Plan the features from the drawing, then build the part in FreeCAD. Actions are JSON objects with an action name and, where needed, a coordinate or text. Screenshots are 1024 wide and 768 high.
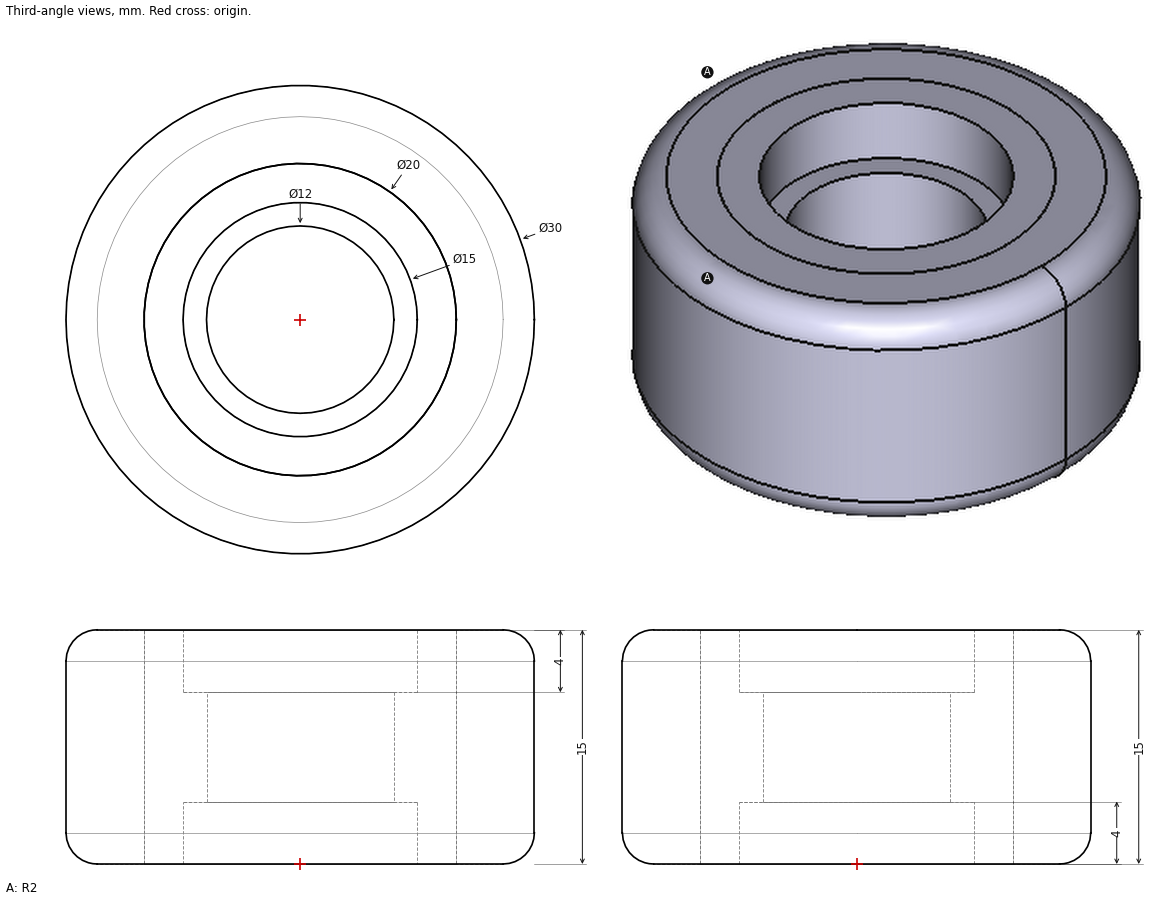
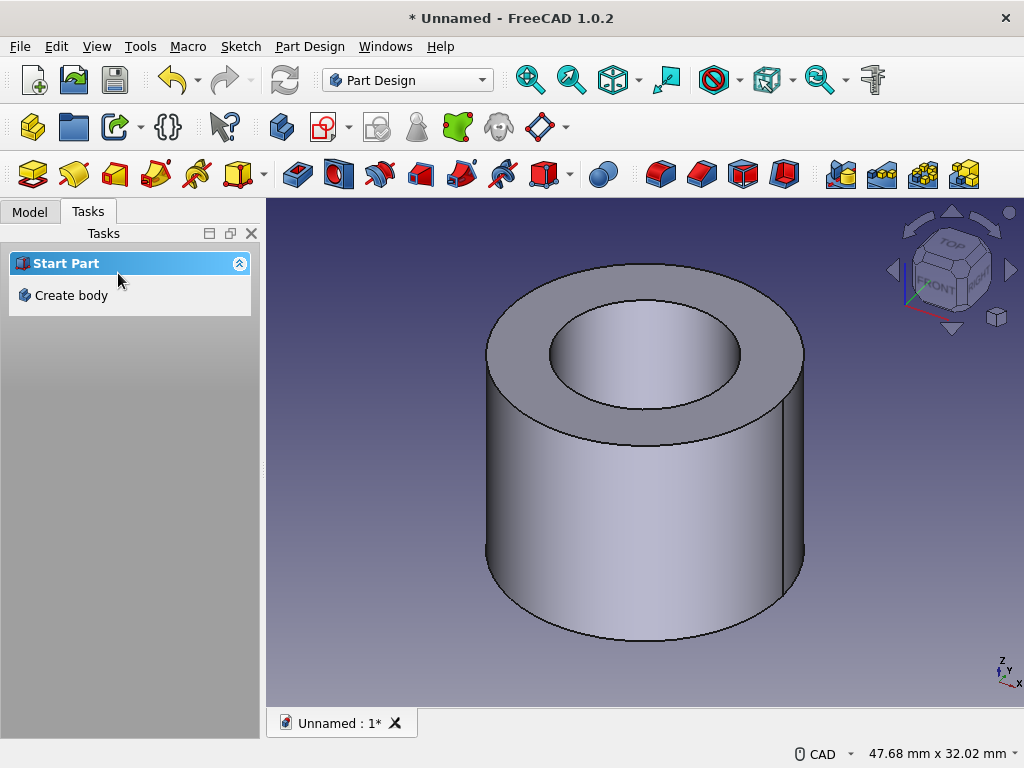
{"action": "left_click", "coordinate": [678, 425]}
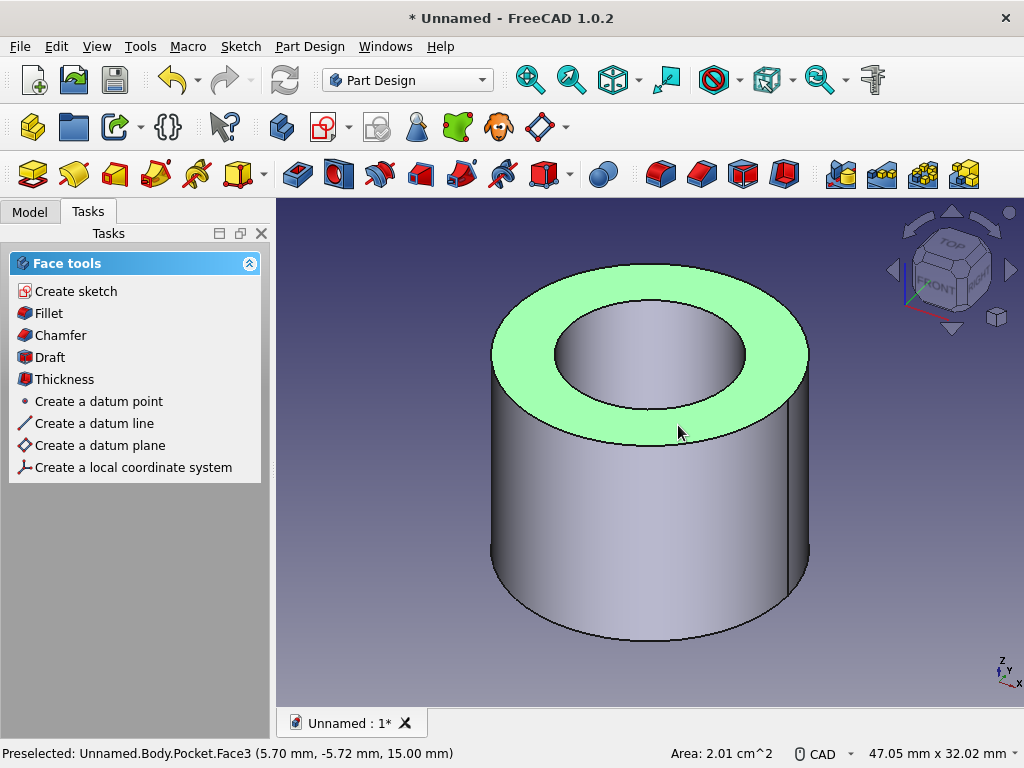
{"action": "left_click", "coordinate": [322, 128]}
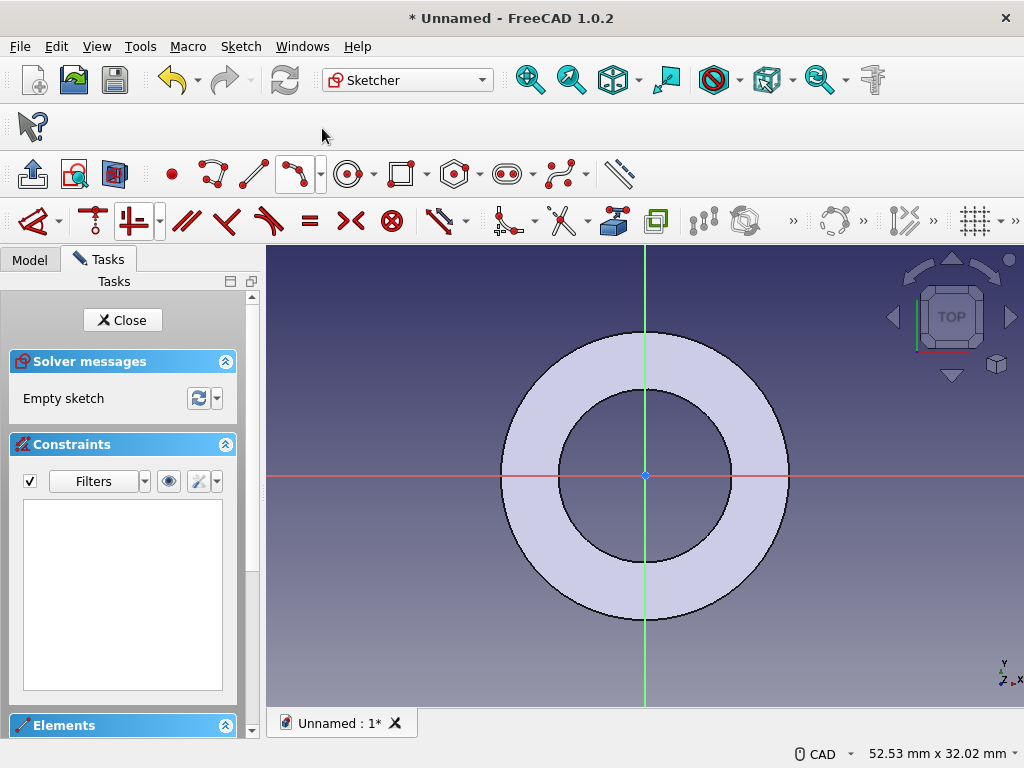
{"action": "key", "text": "g c"}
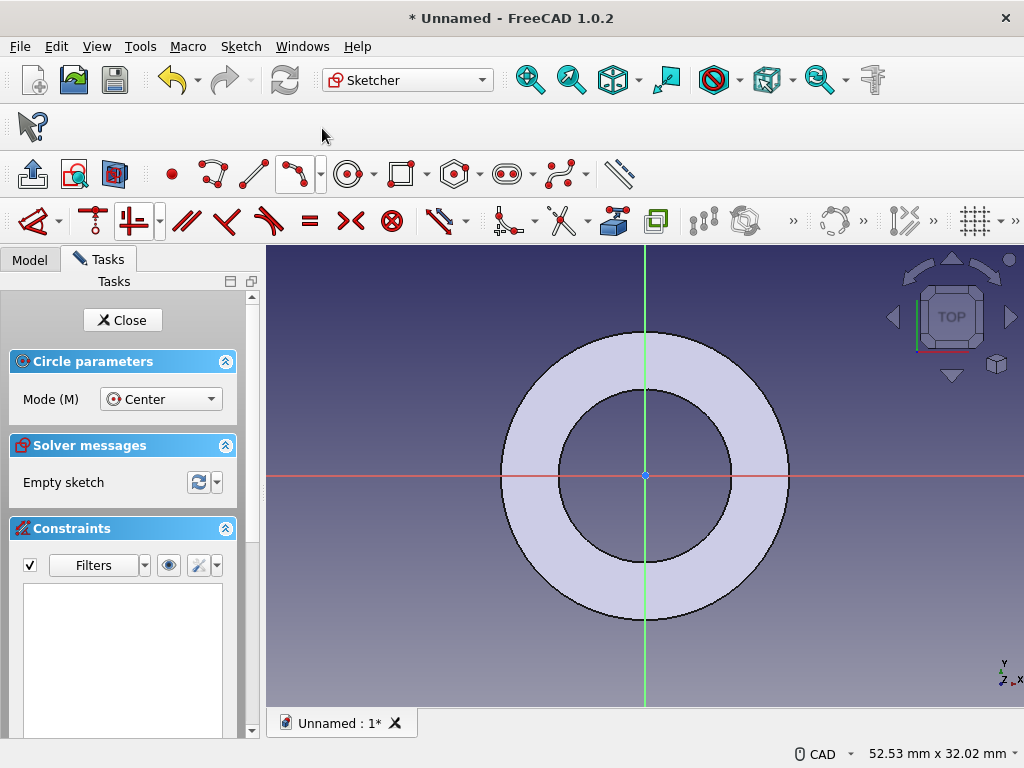
{"action": "left_click", "coordinate": [645, 476]}
{"action": "mouse_move", "coordinate": [722, 399]}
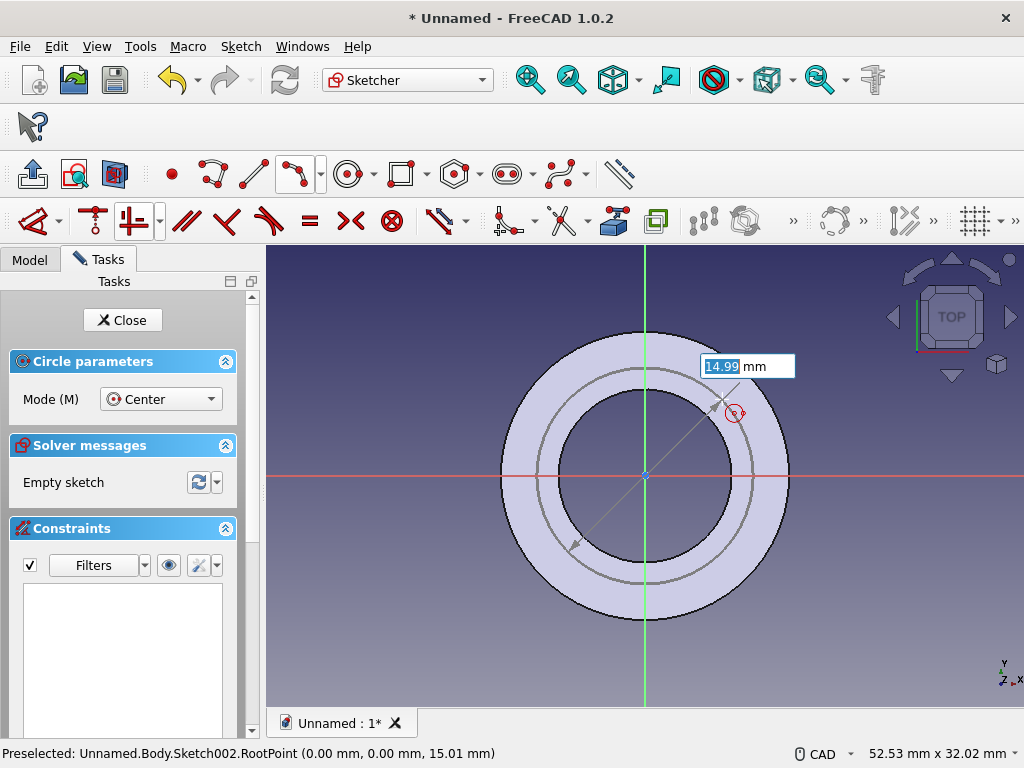
{"action": "type", "text": "15"}
{"action": "key", "text": "Return"}
{"action": "key", "text": "Escape"}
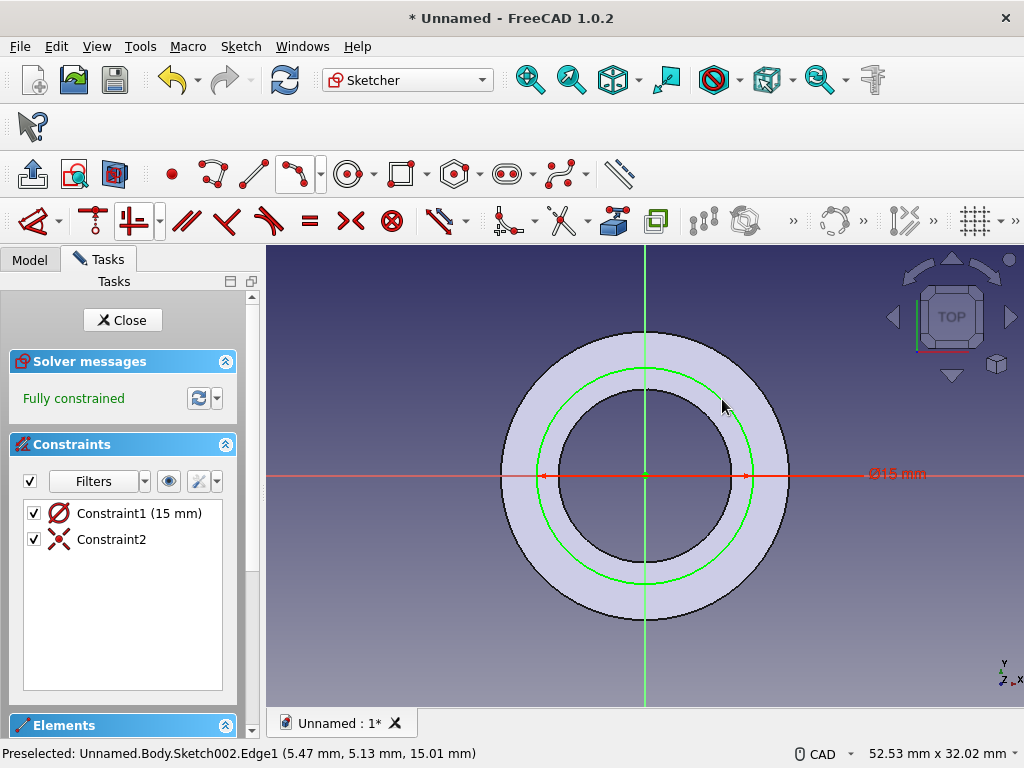
{"action": "left_click", "coordinate": [123, 320]}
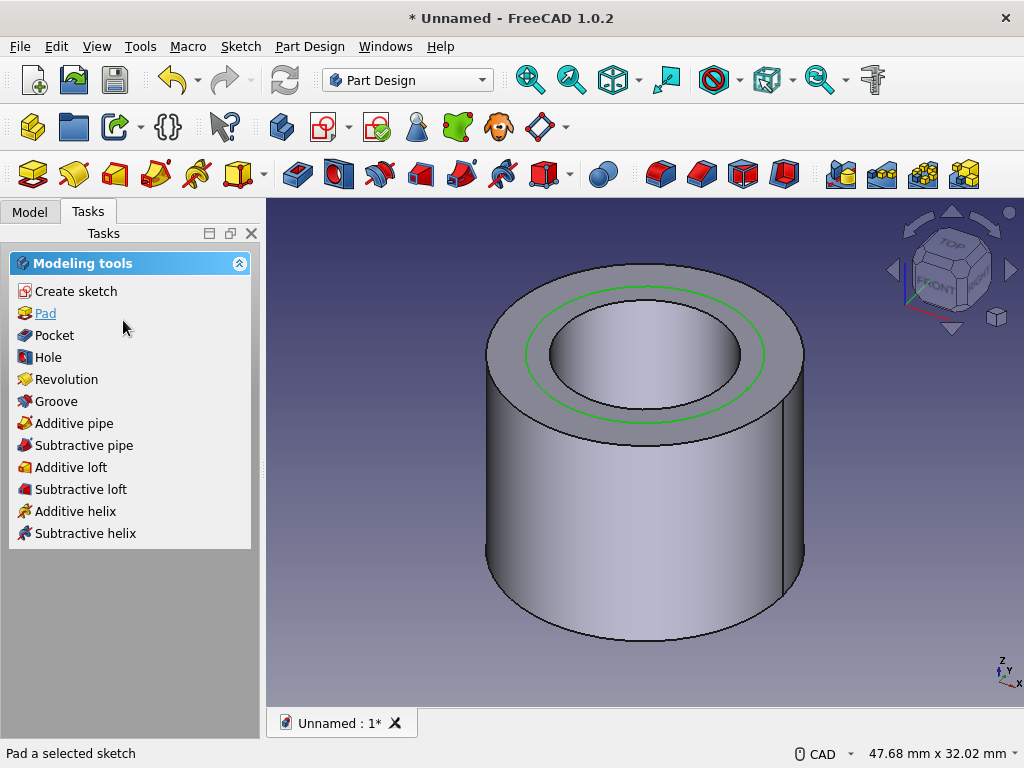
{"action": "left_click", "coordinate": [298, 174]}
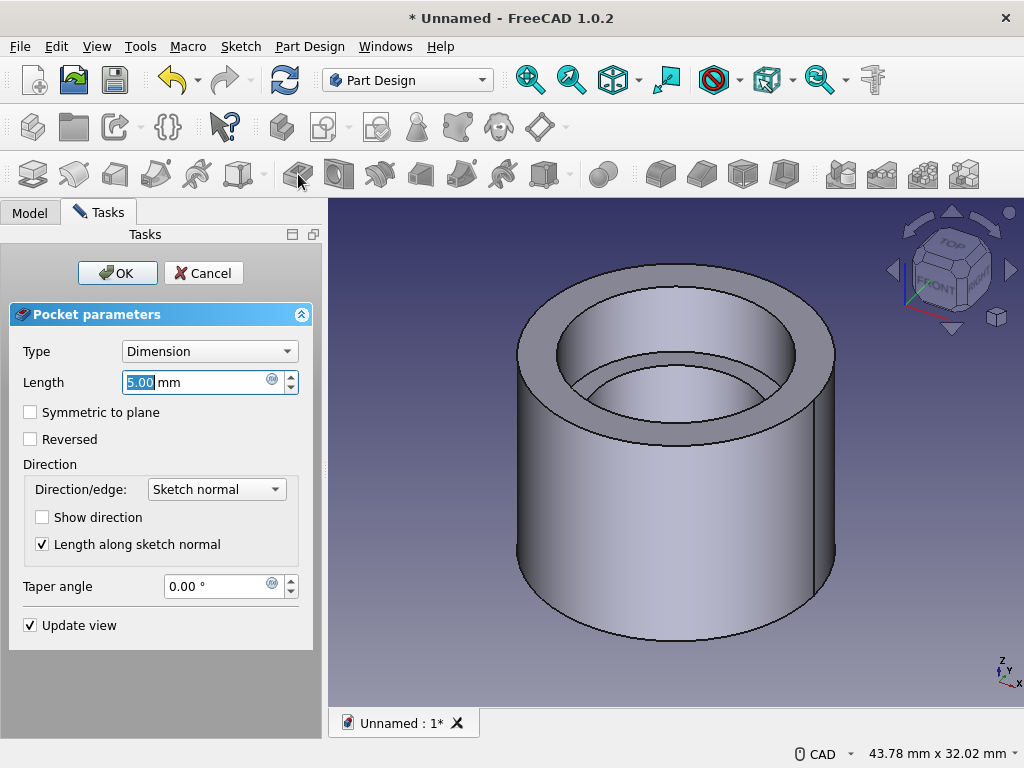
{"action": "type", "text": "4"}
{"action": "key", "text": "Tab"}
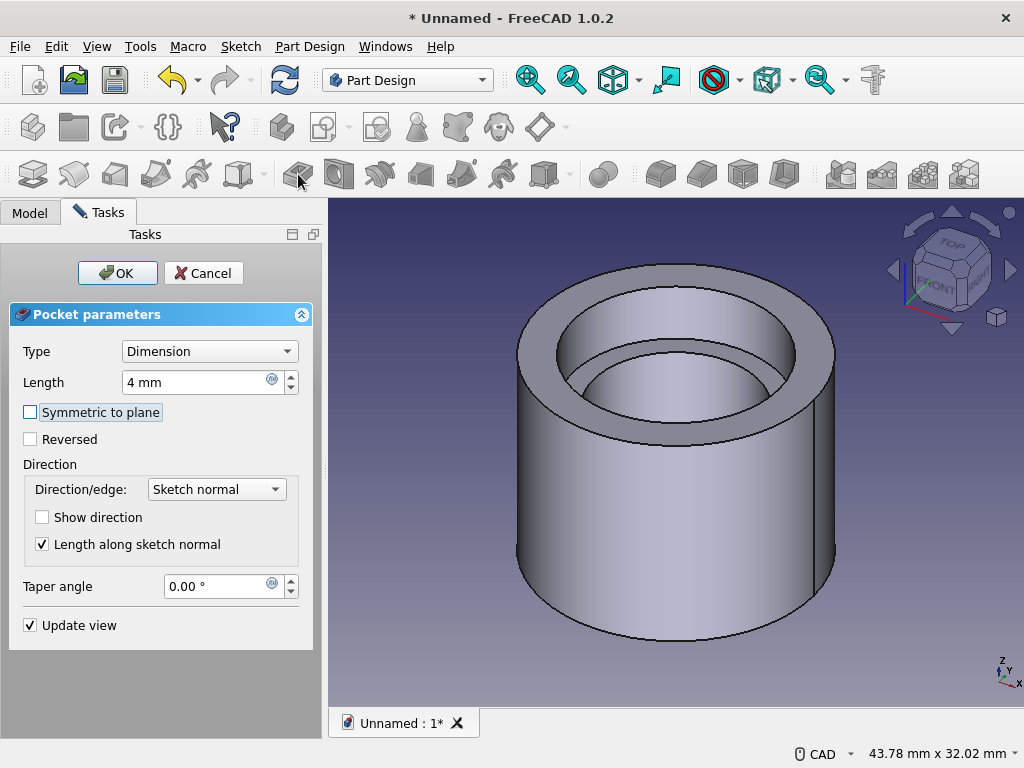
{"action": "left_click", "coordinate": [118, 273]}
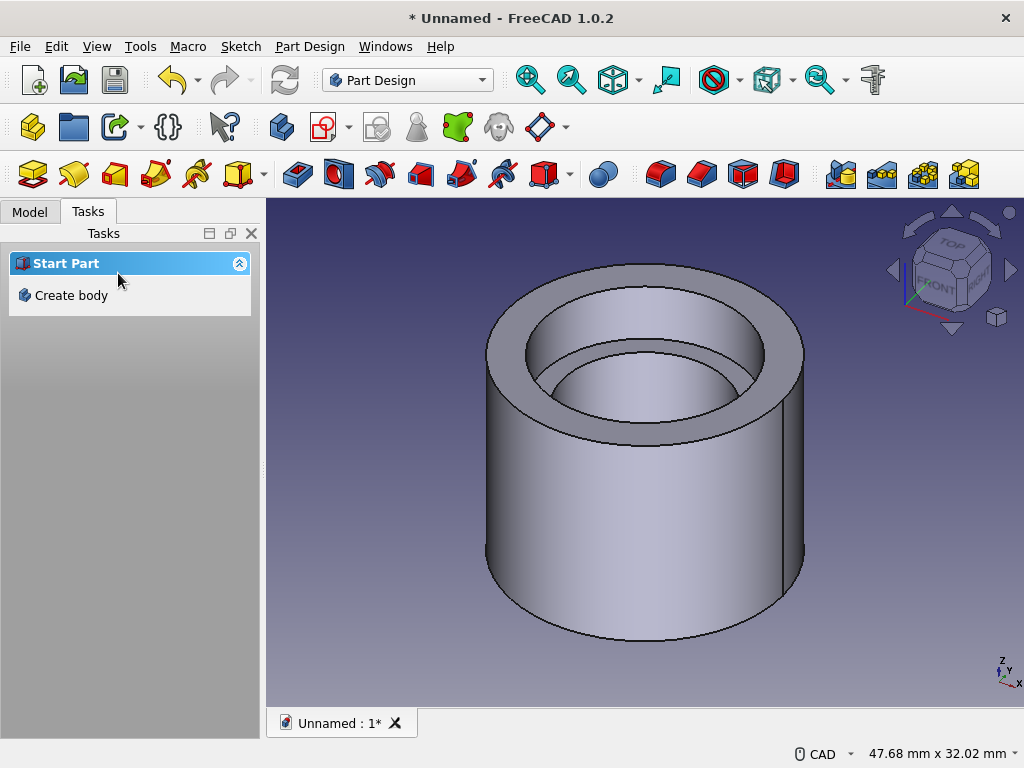
{"action": "left_click", "coordinate": [30, 212]}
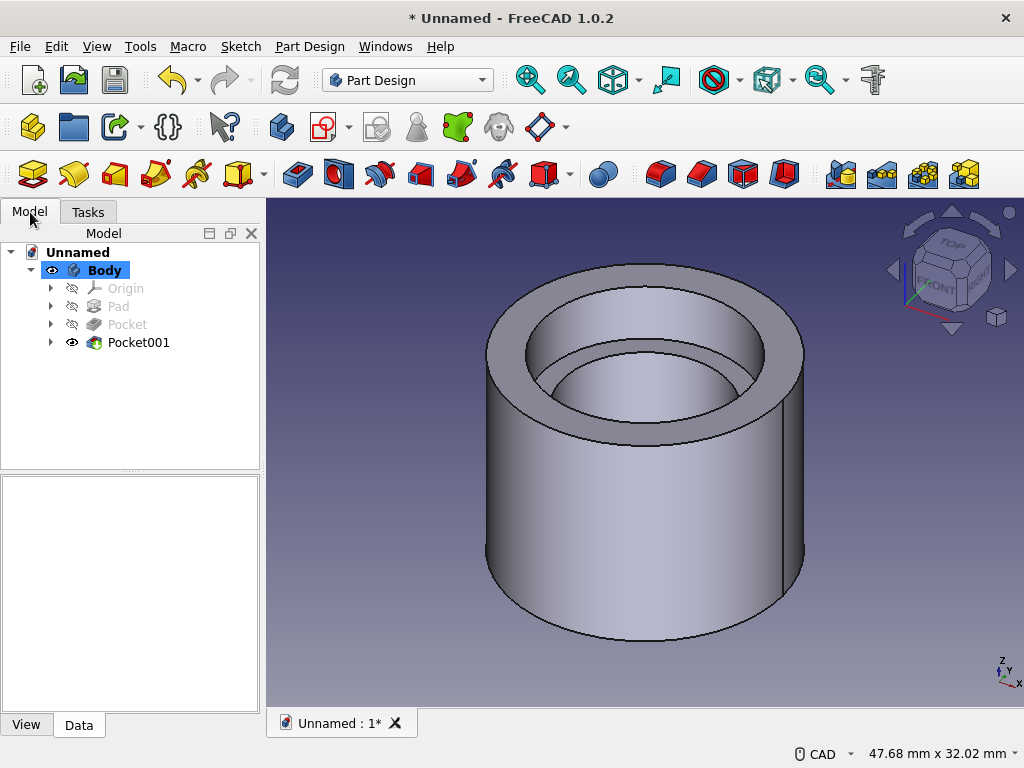
{"action": "left_click", "coordinate": [51, 288]}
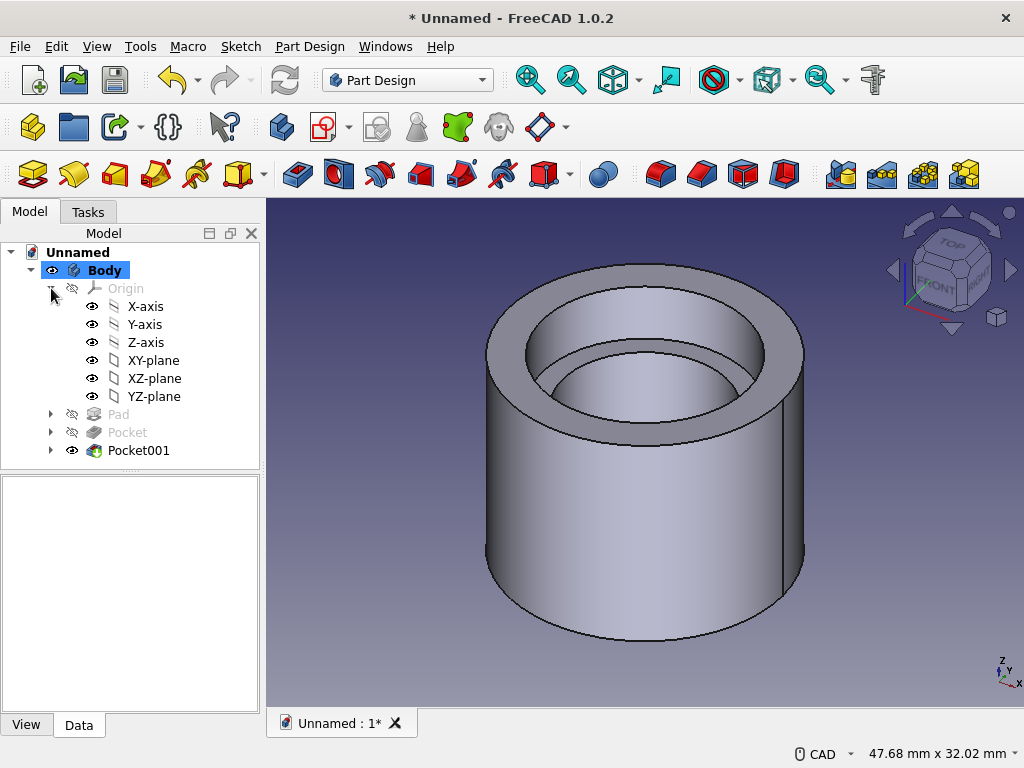
{"action": "left_click", "coordinate": [137, 360]}